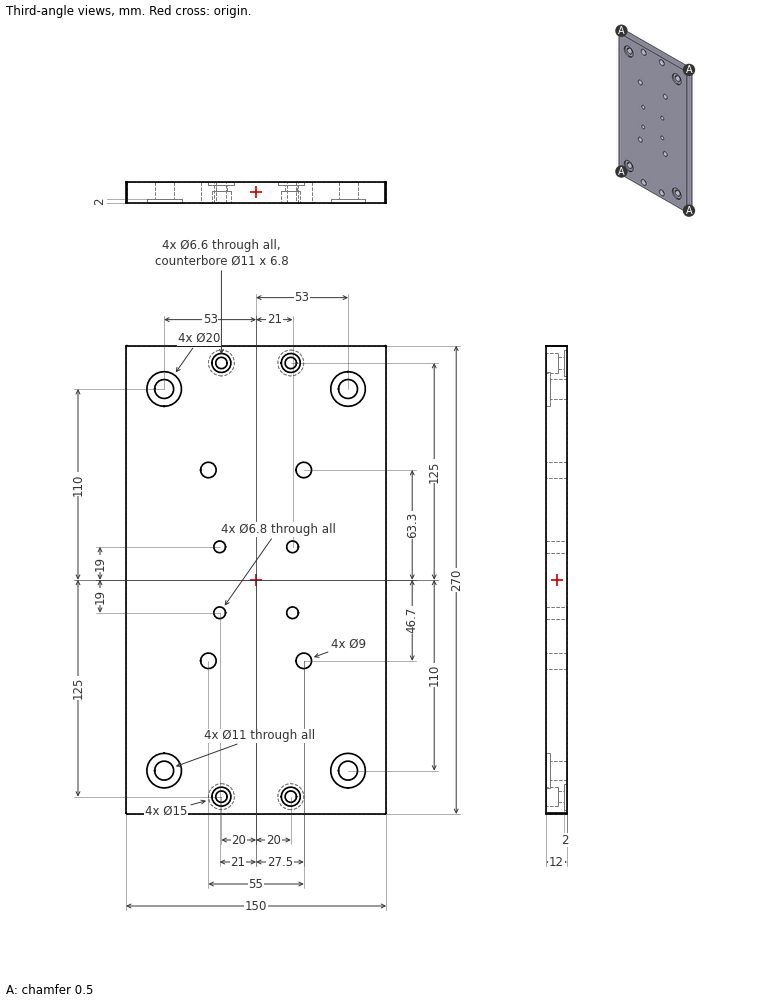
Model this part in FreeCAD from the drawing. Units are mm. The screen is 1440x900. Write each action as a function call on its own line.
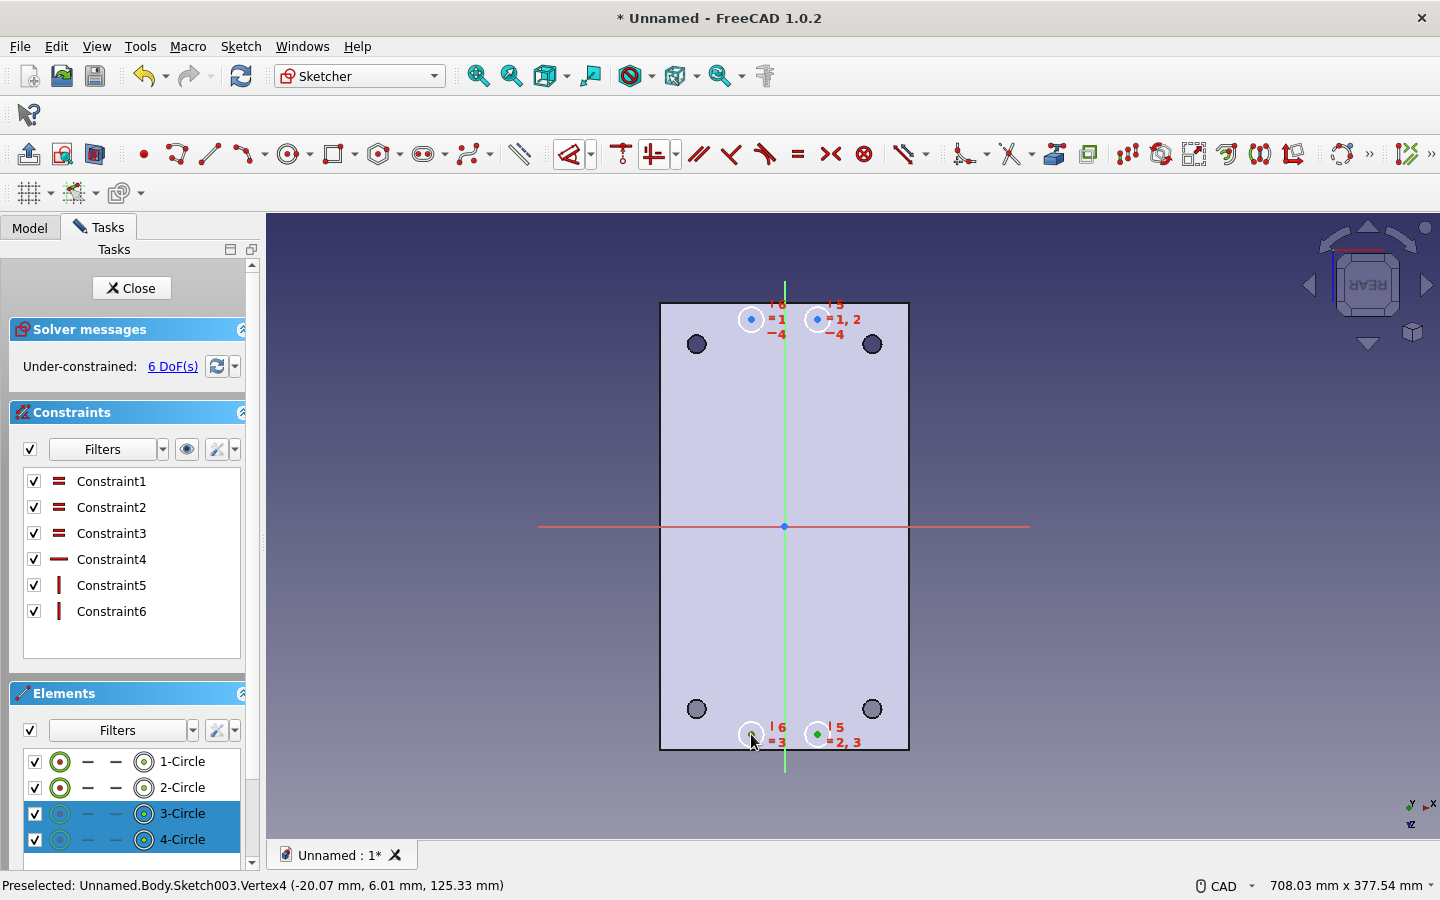
key(h)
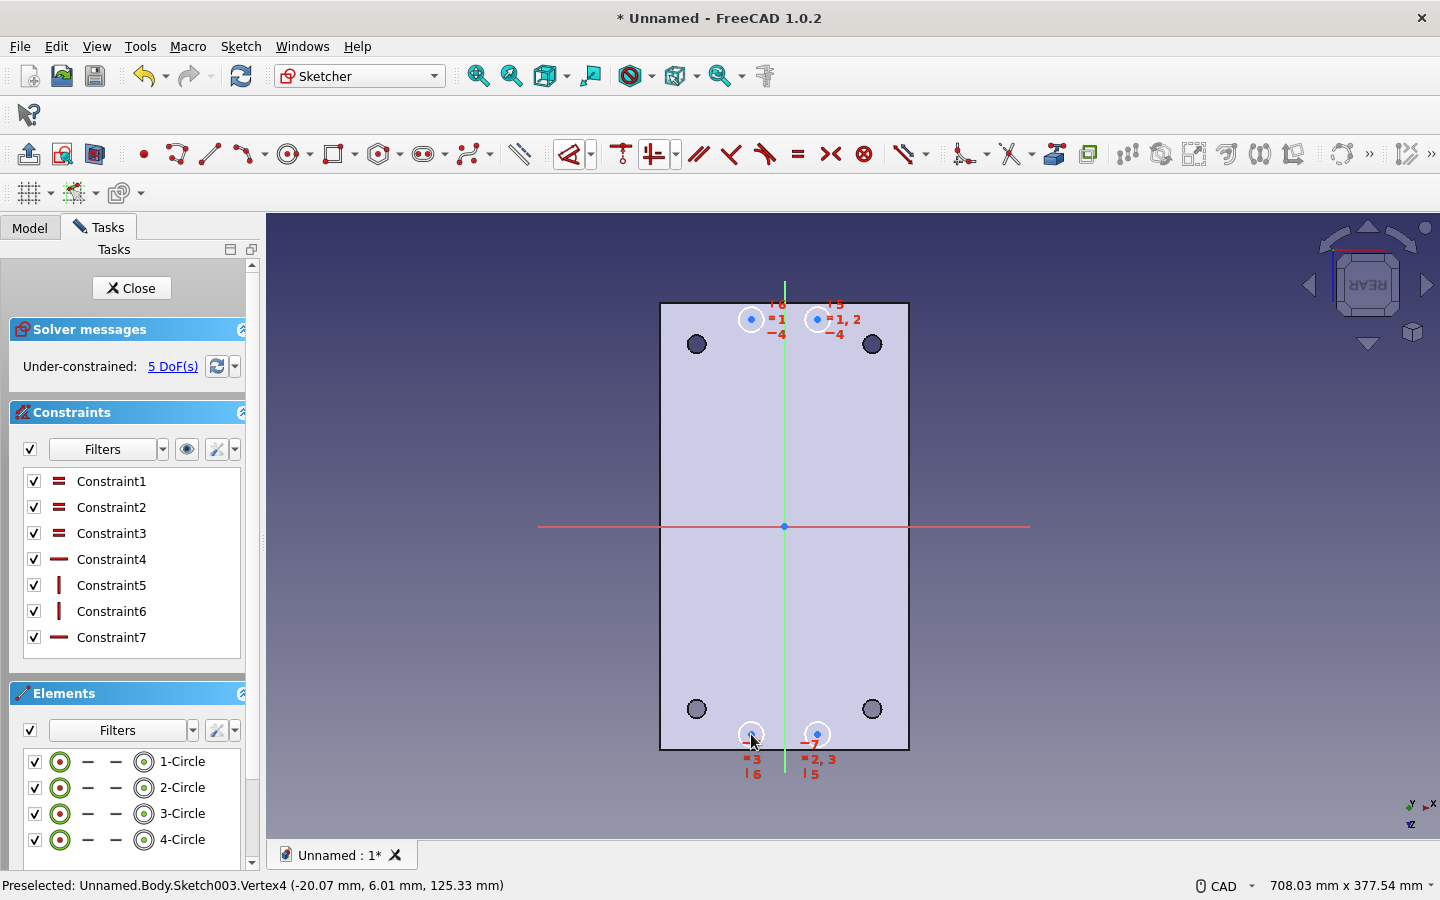
scroll(760, 311, up, 3)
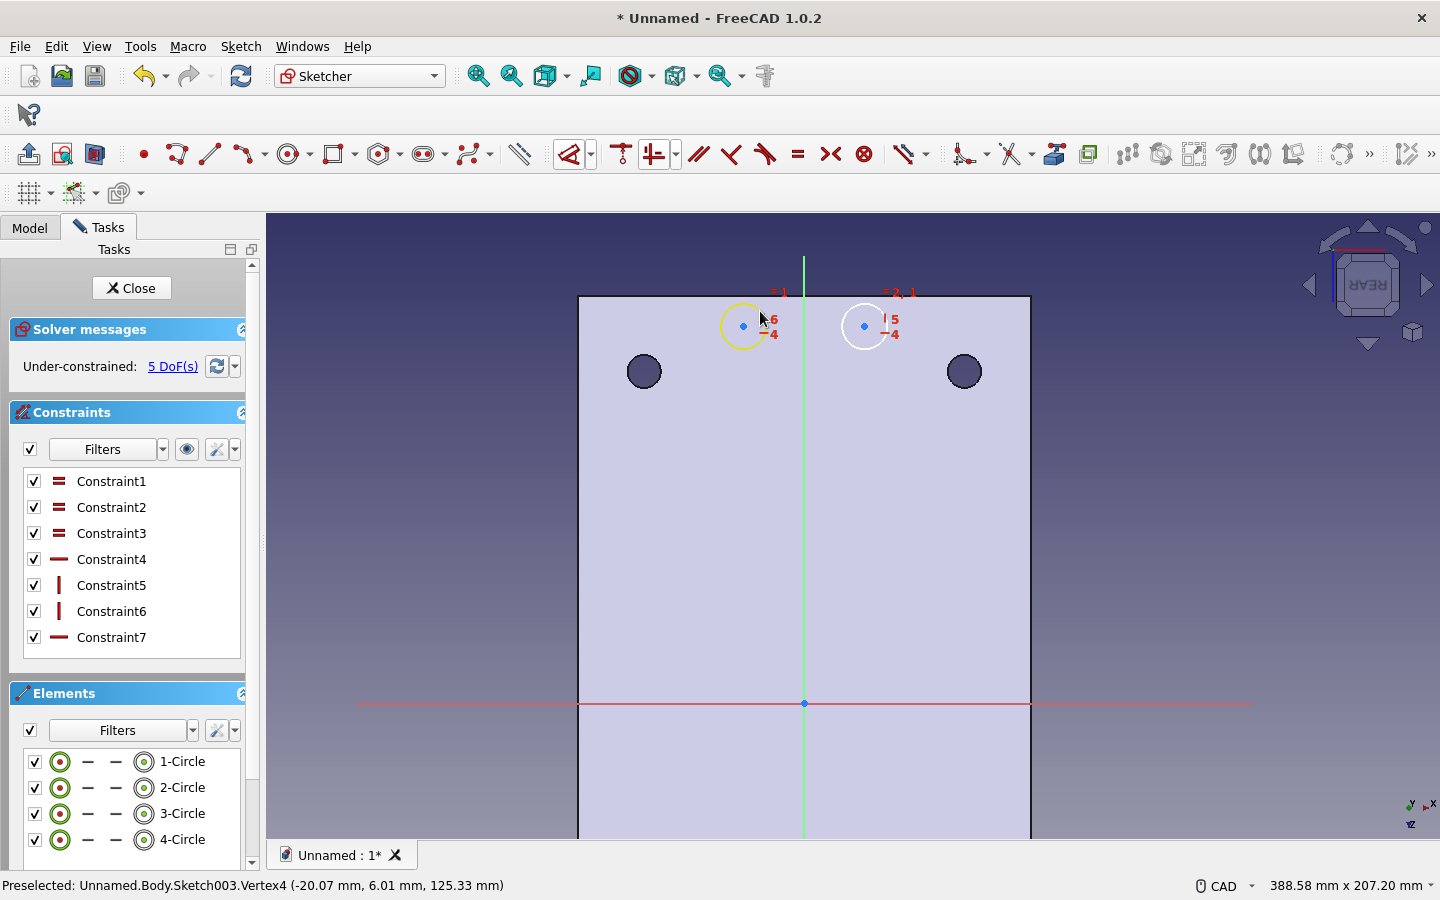
click(728, 311)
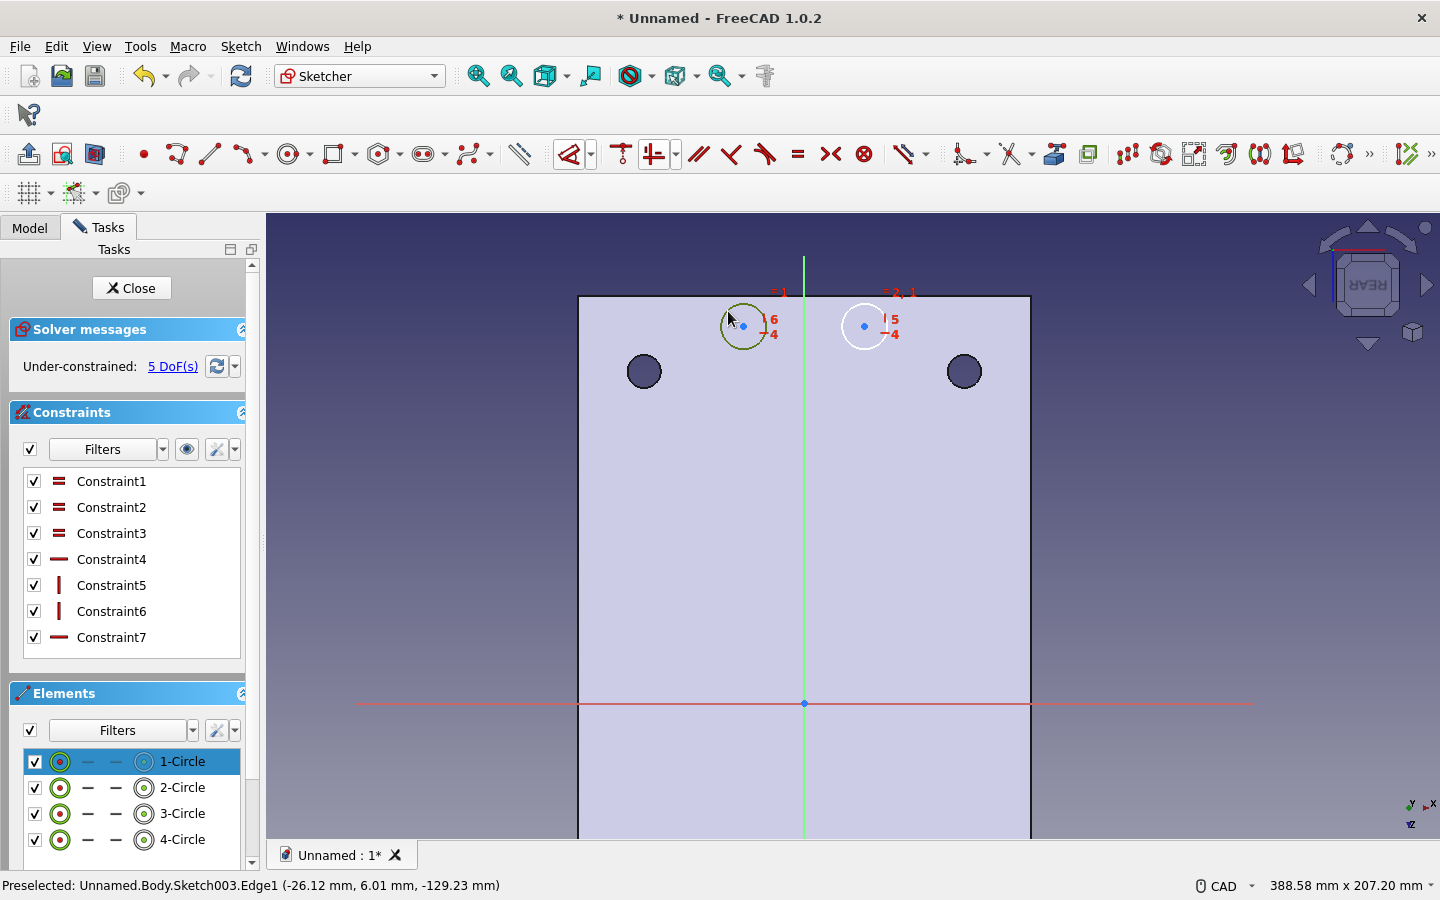
key(k)
key(o)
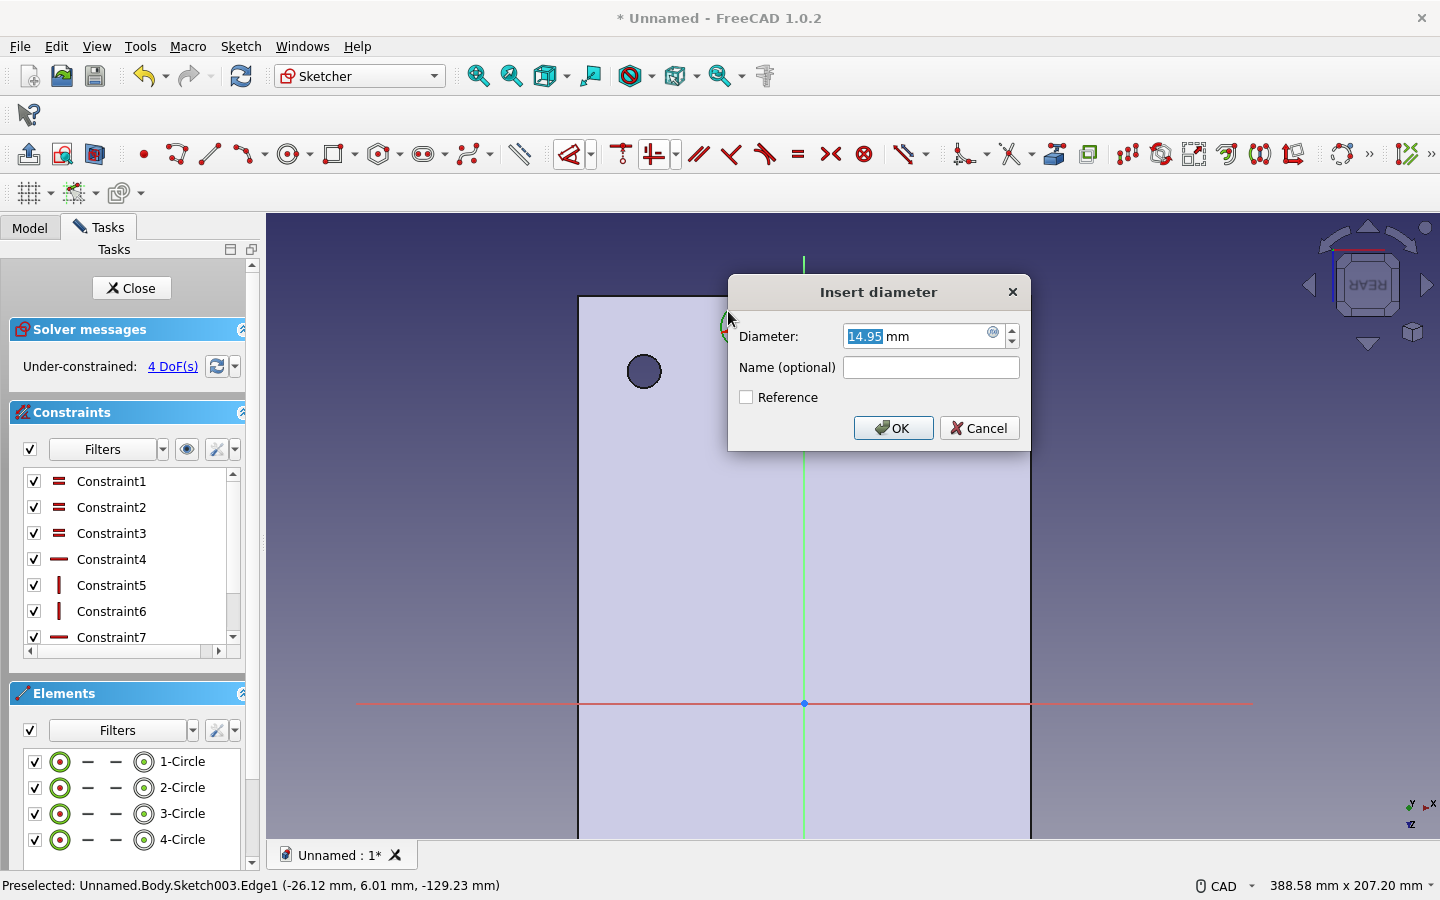
text(15)
key(Return)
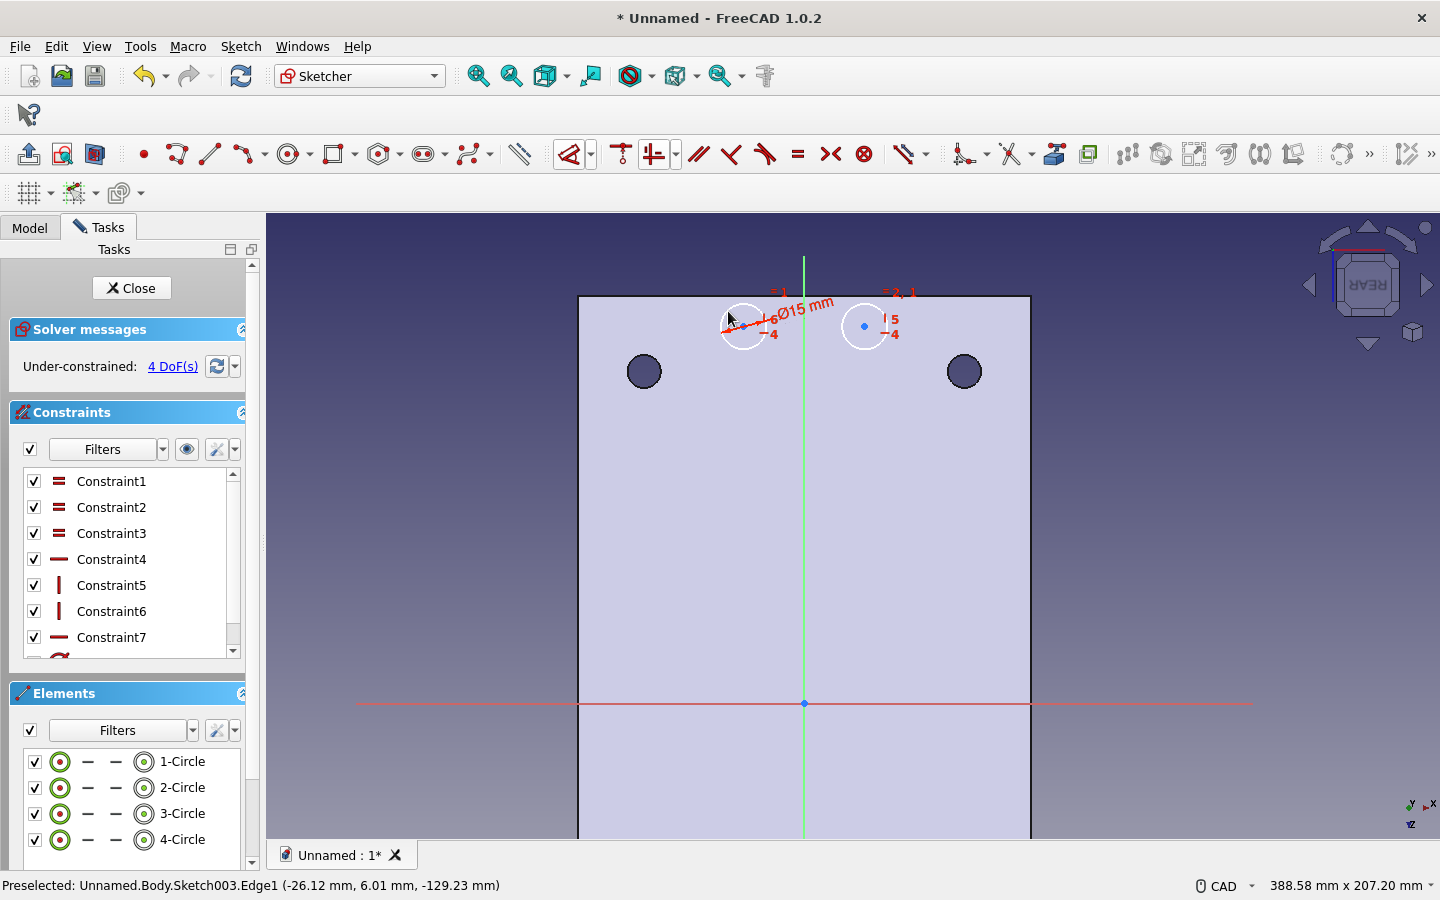
click(744, 327)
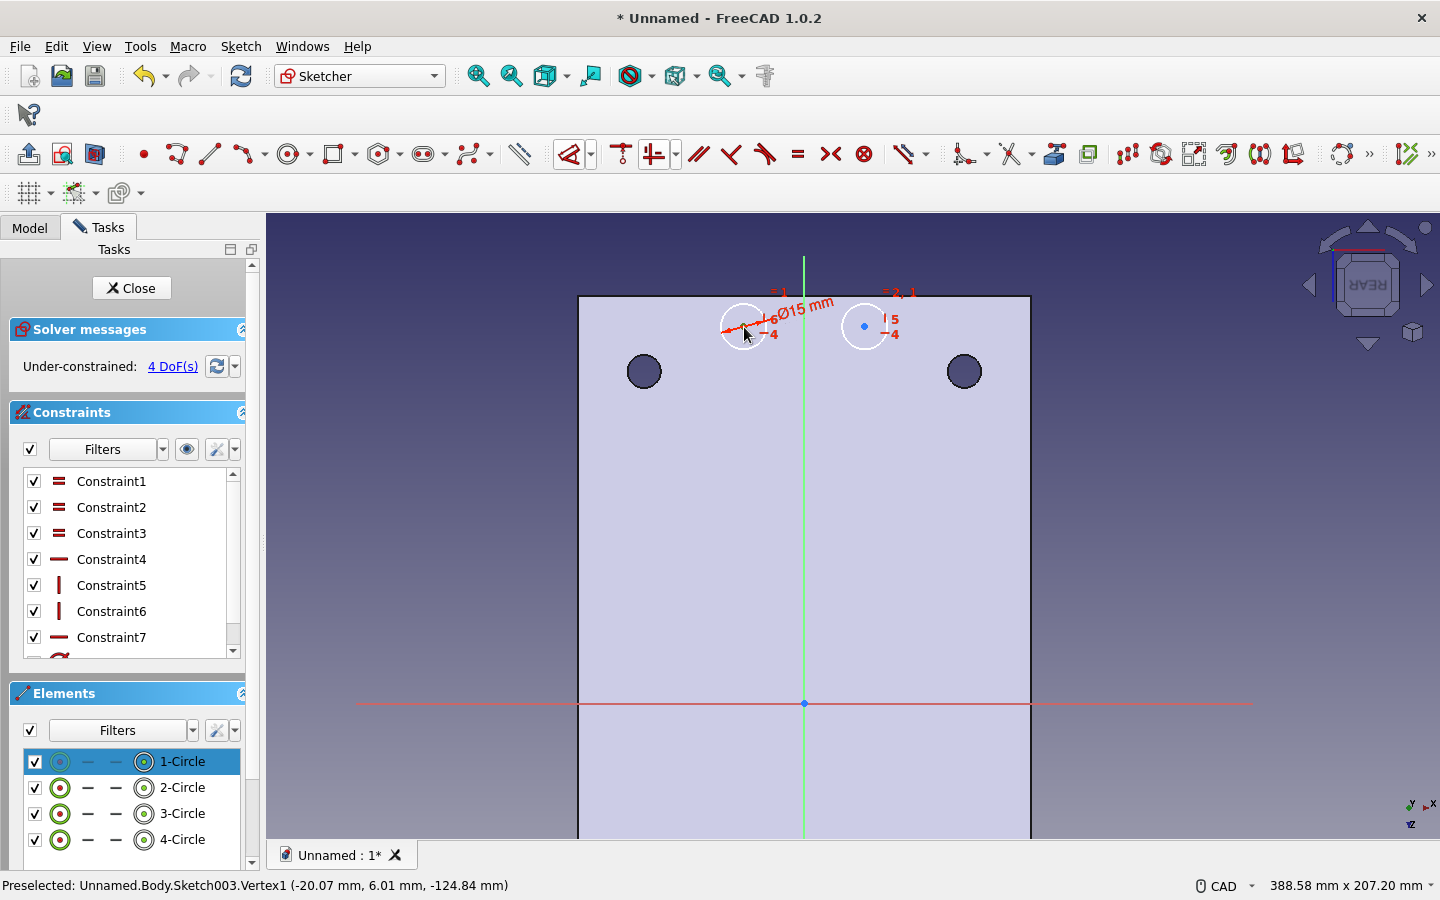
key(l)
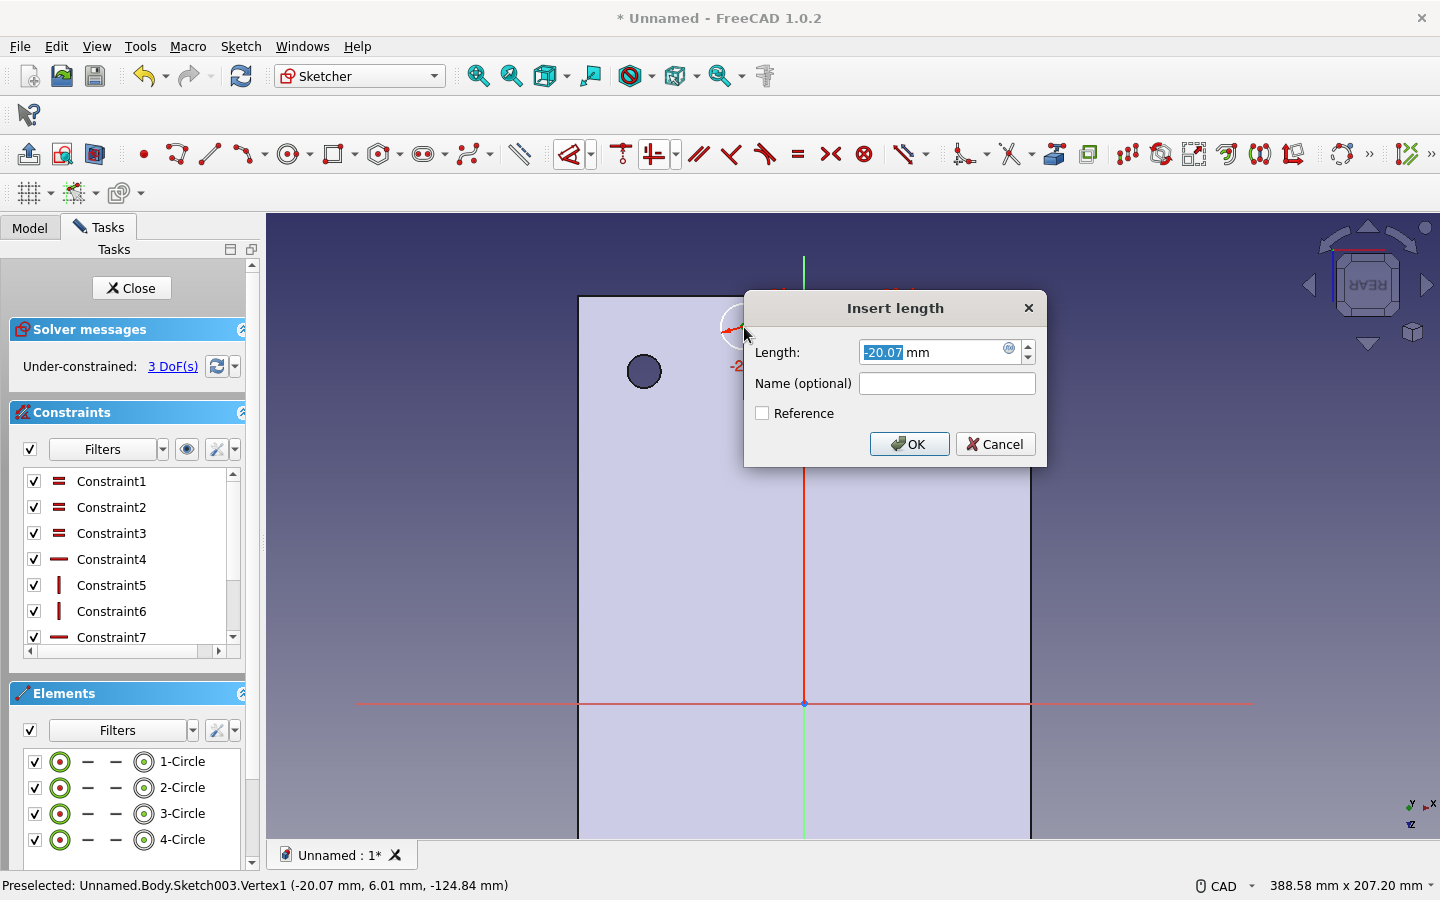
text(-20)
key(Return)